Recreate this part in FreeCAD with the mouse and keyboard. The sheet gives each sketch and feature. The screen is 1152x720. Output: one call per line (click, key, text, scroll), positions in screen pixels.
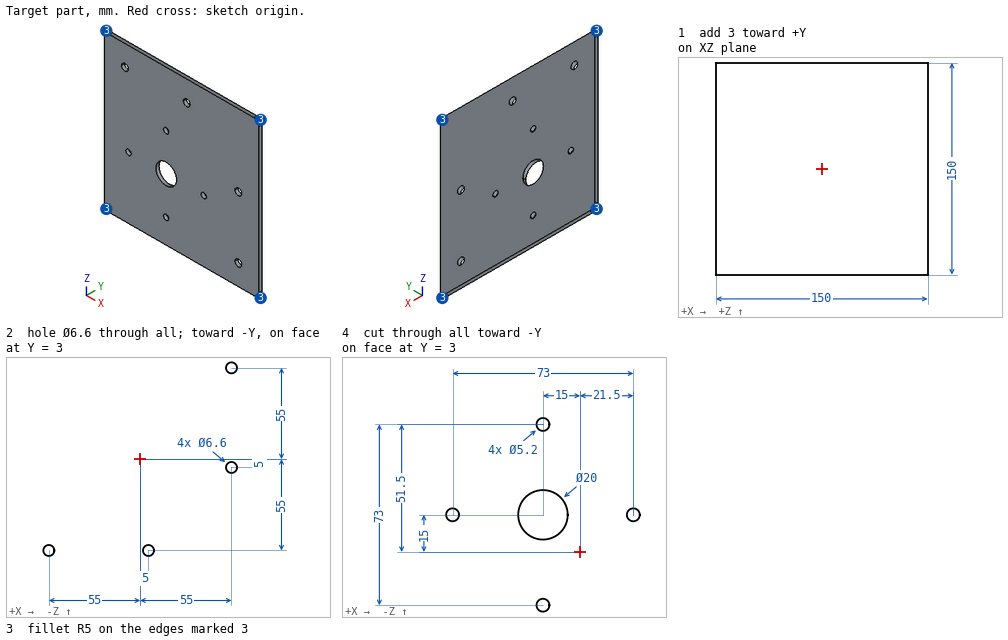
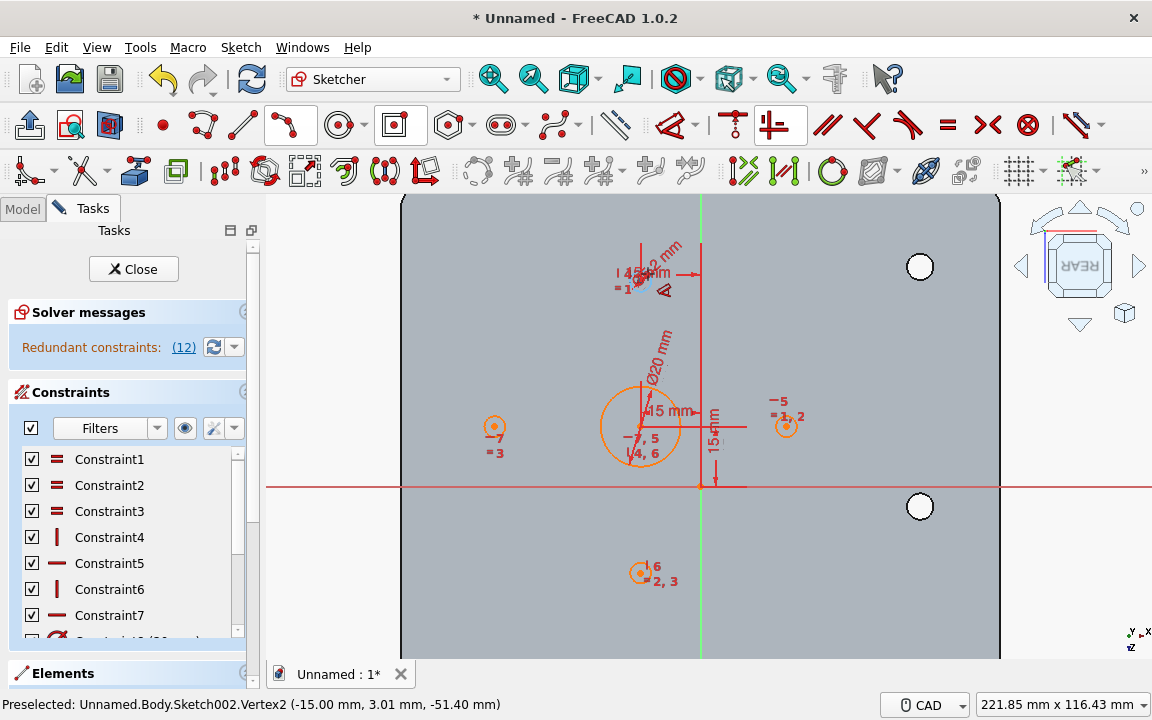
click(641, 573)
click(675, 325)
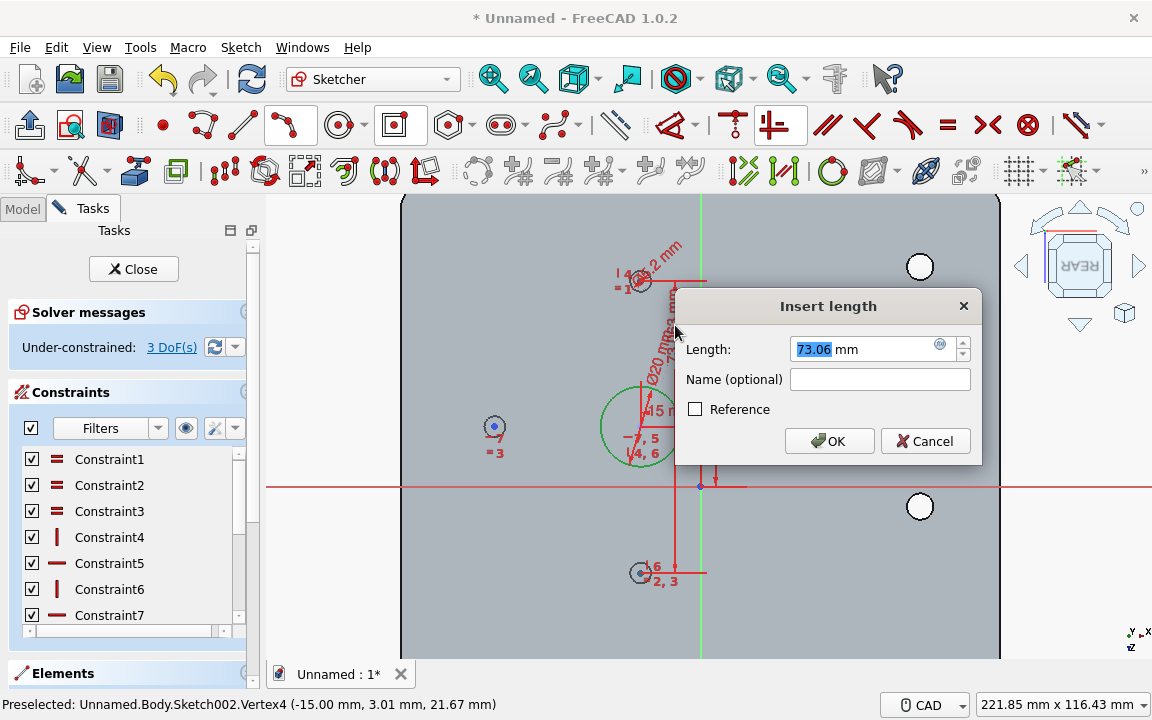
text(73)
key(Return)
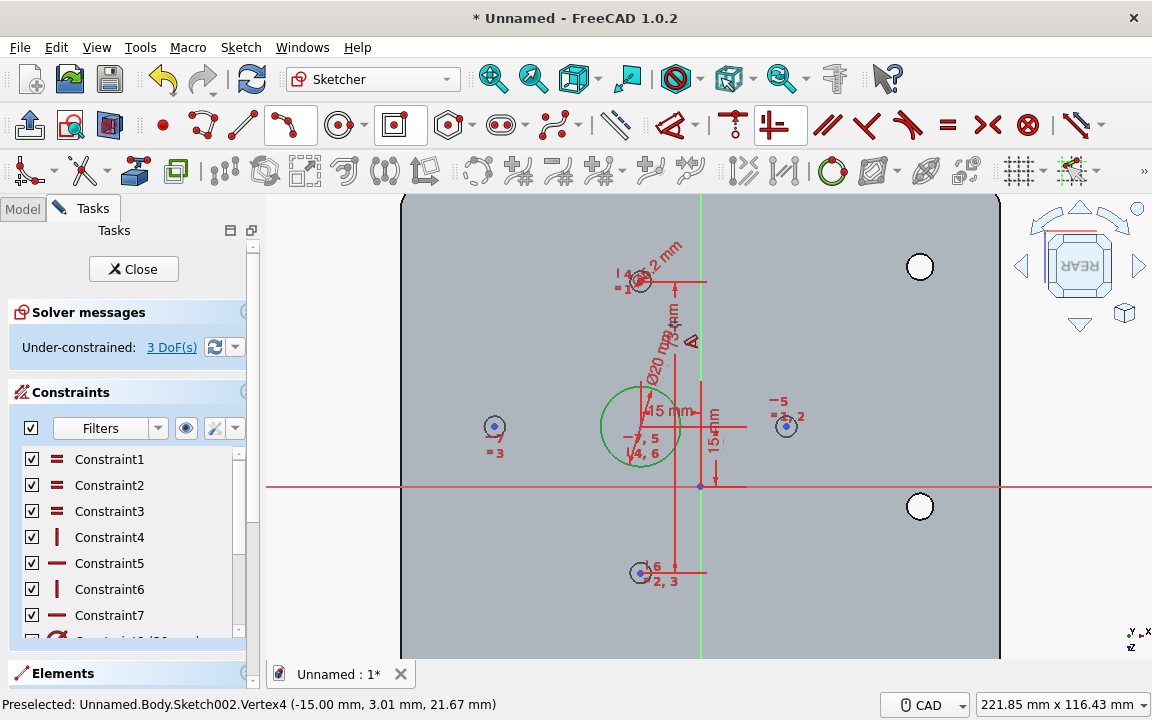
click(786, 427)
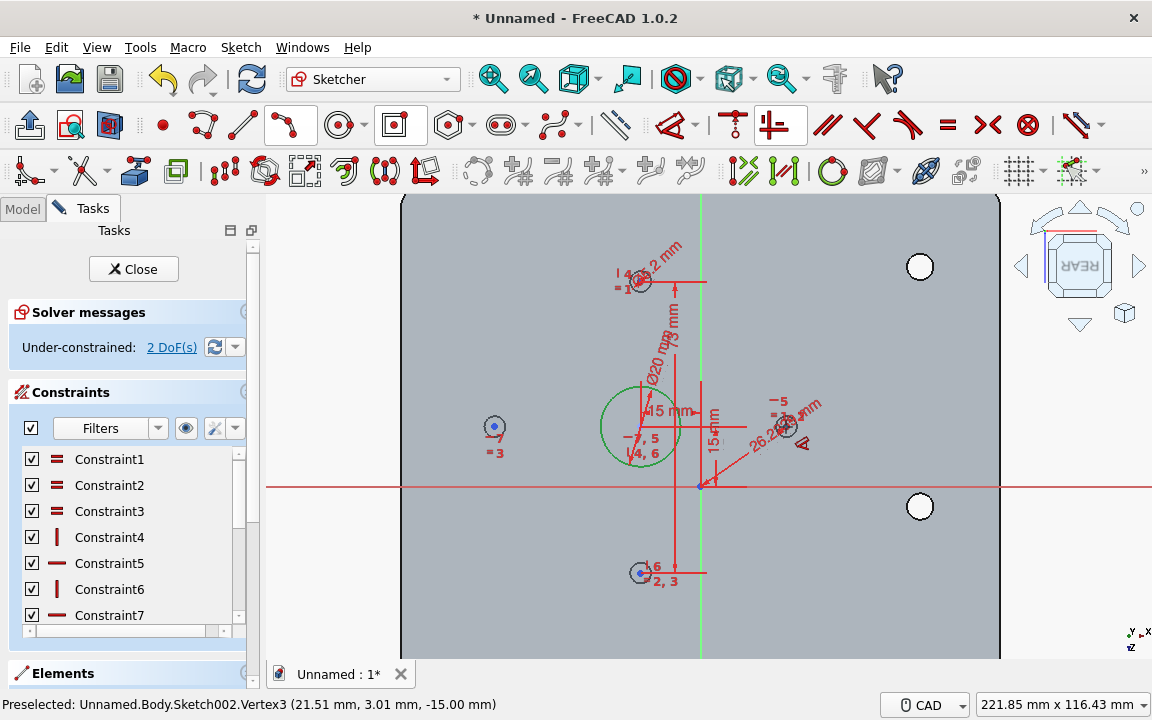
click(495, 427)
click(574, 461)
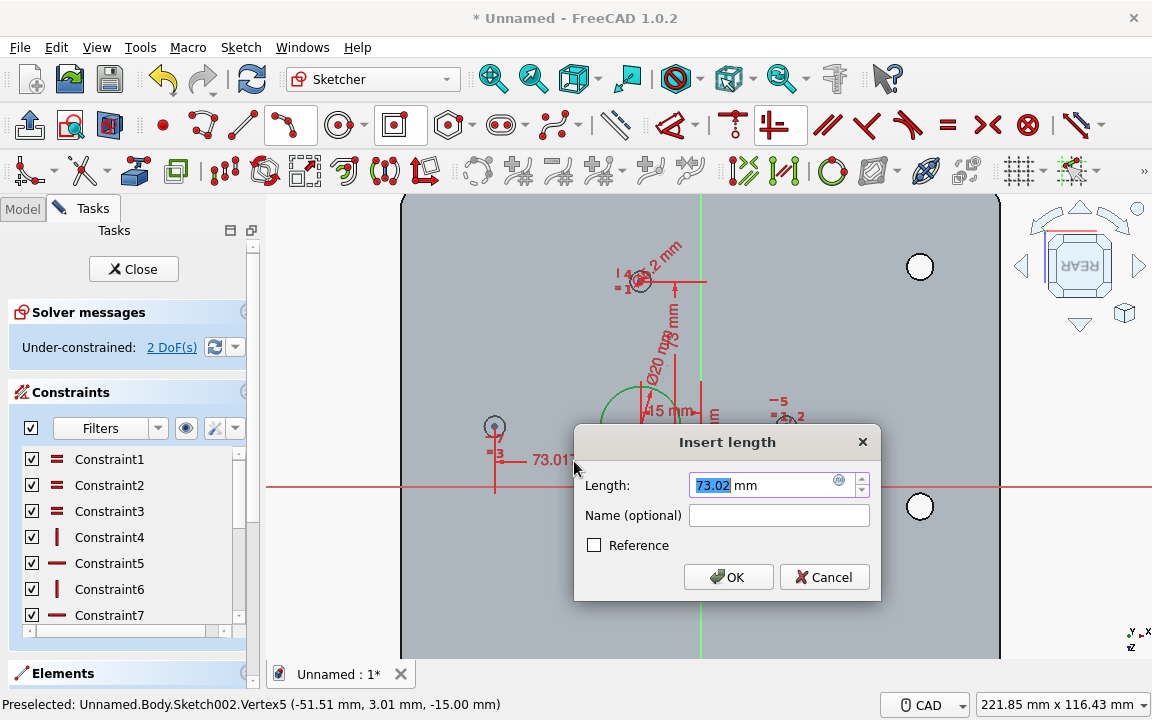
text(73)
key(Return)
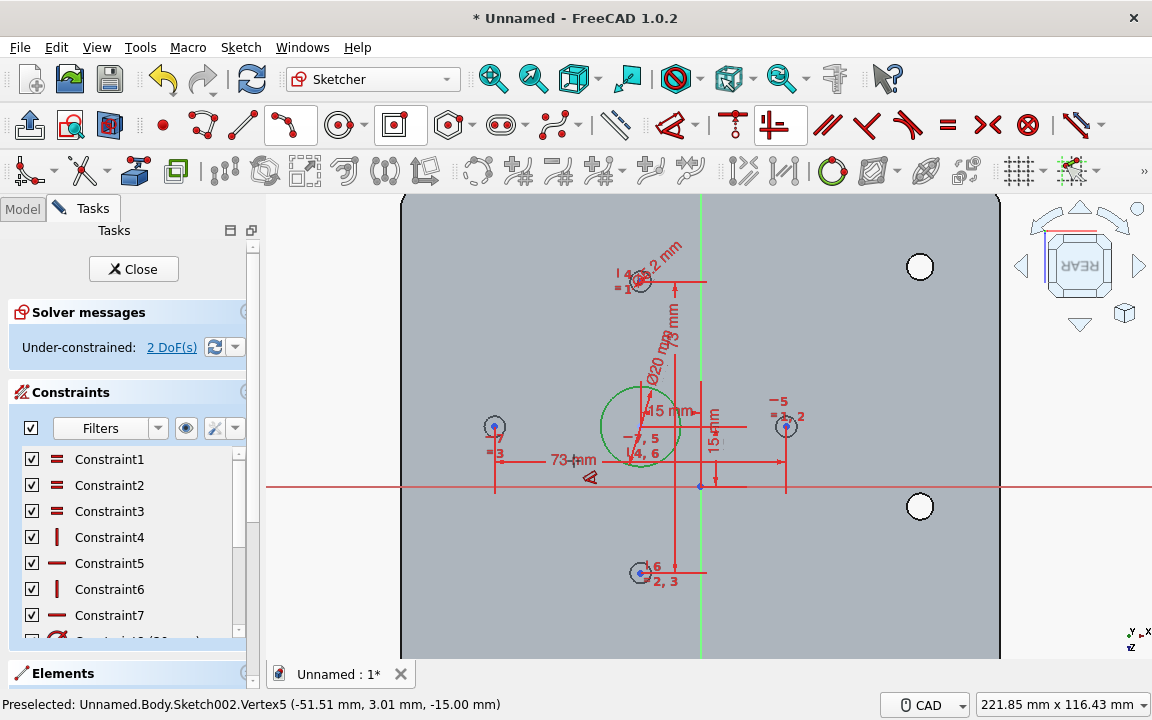
click(641, 282)
click(735, 384)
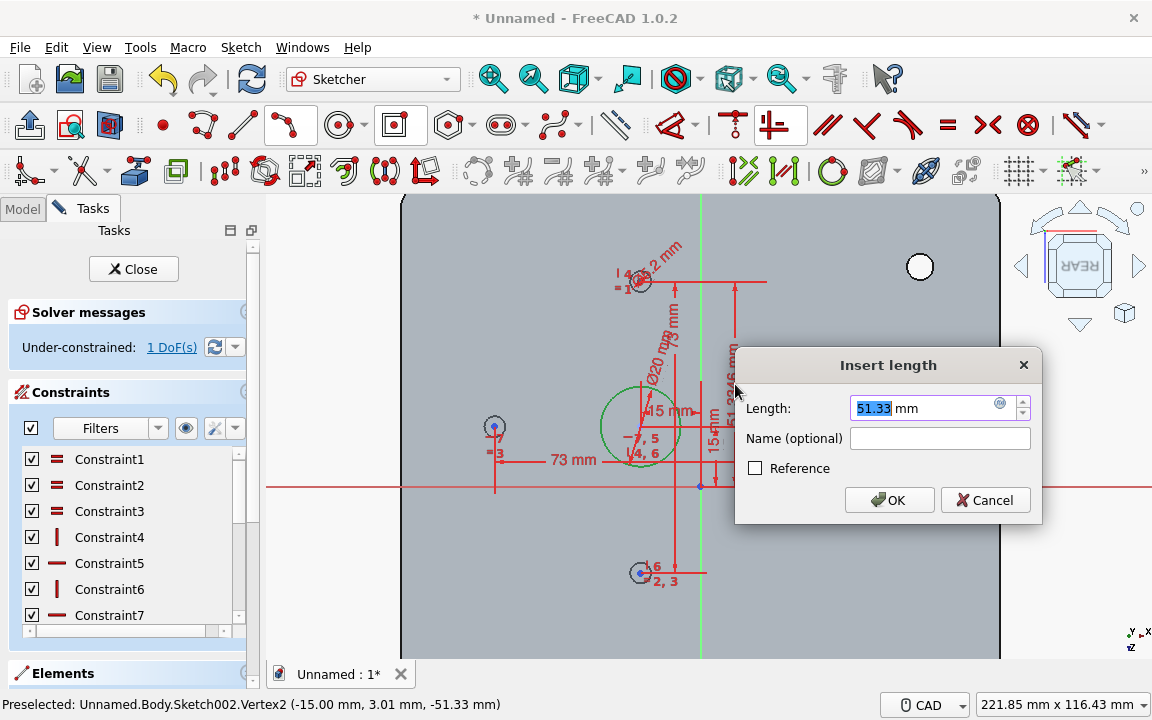
text(51.5)
key(Return)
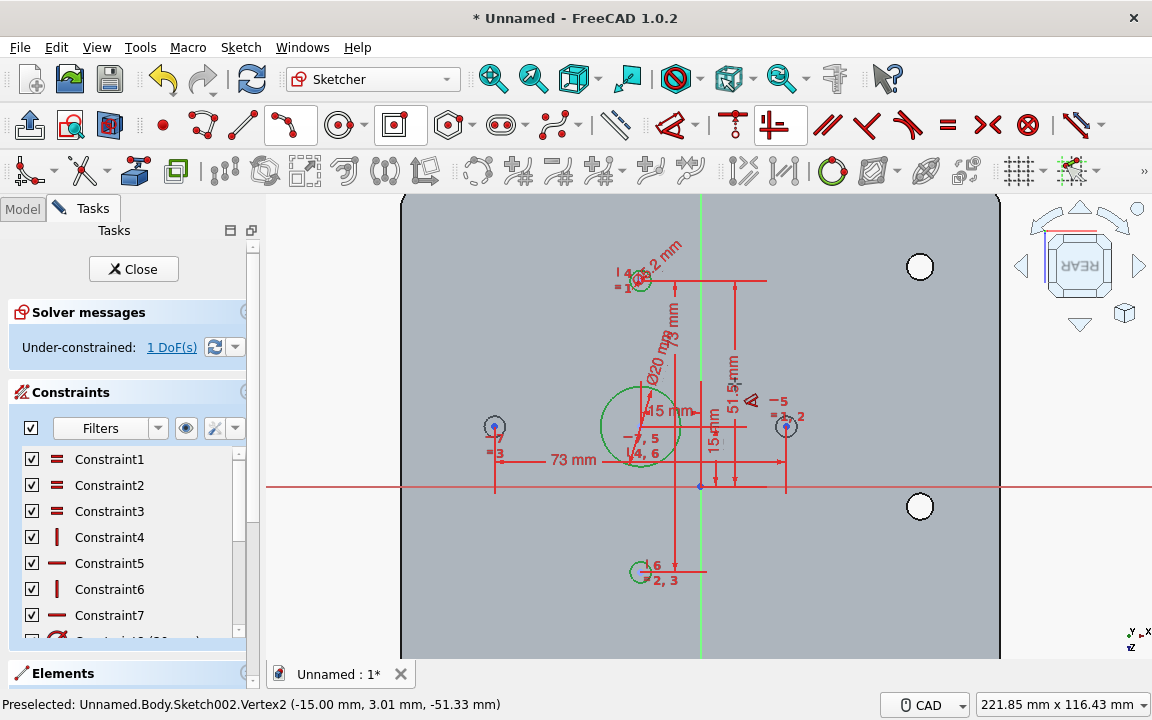
click(786, 427)
click(743, 521)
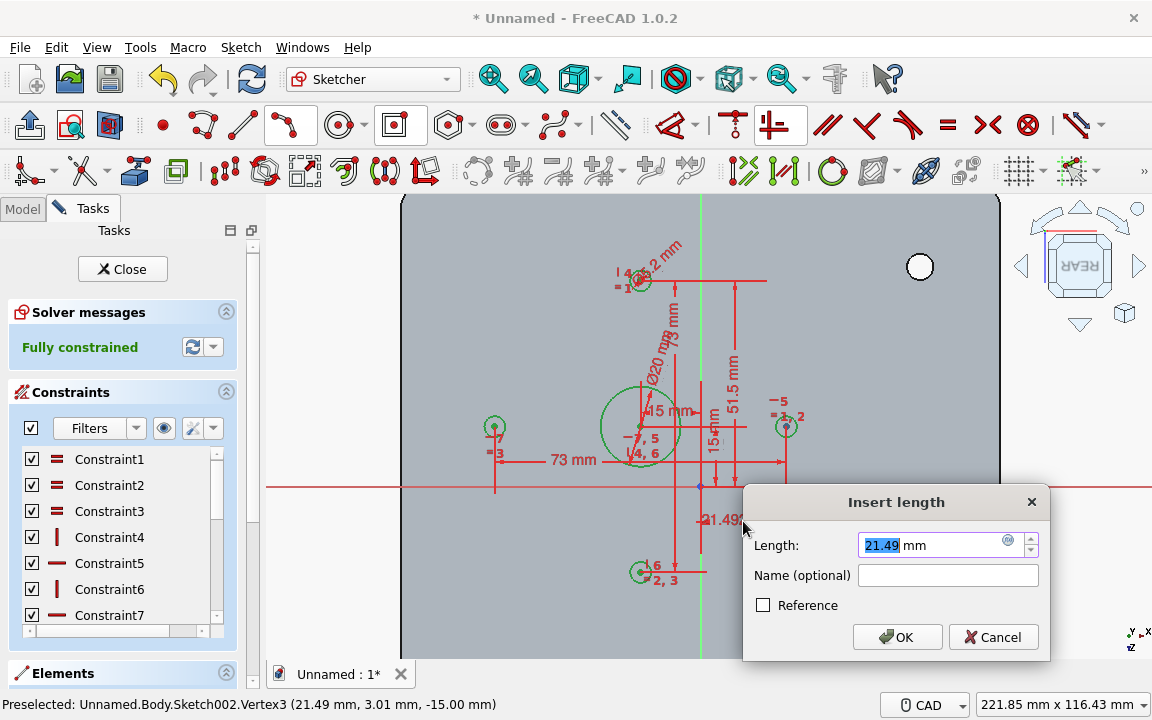
text(21.5)
key(Return)
key(Escape)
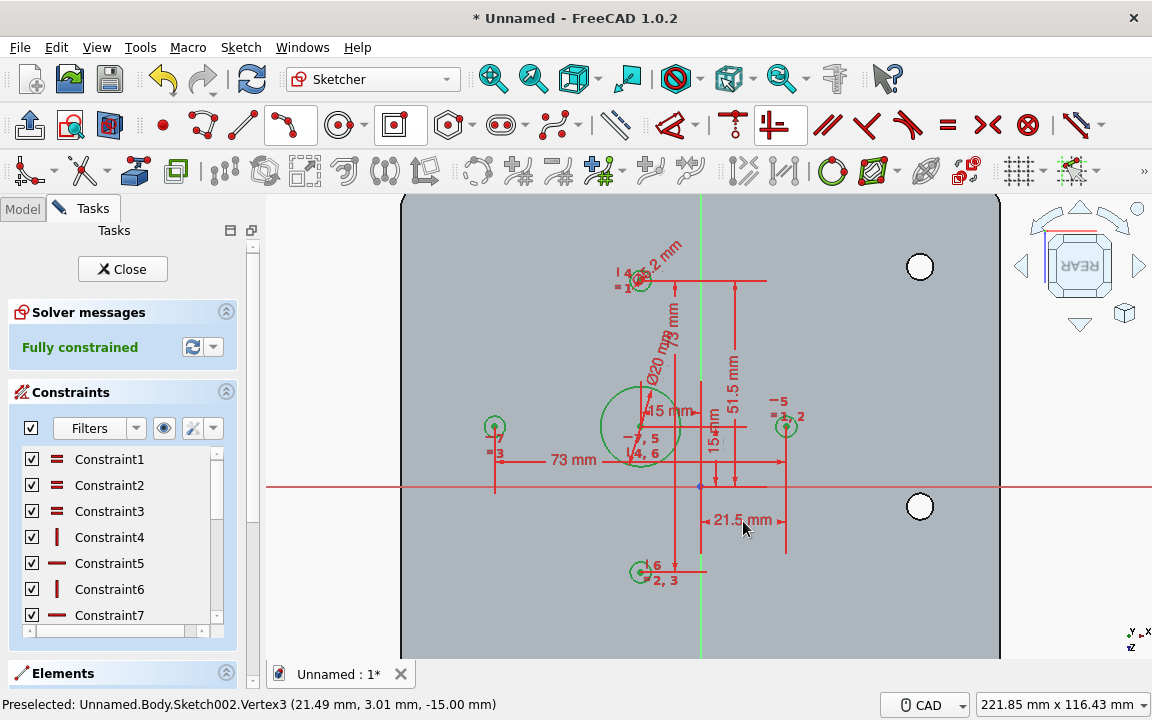
click(123, 269)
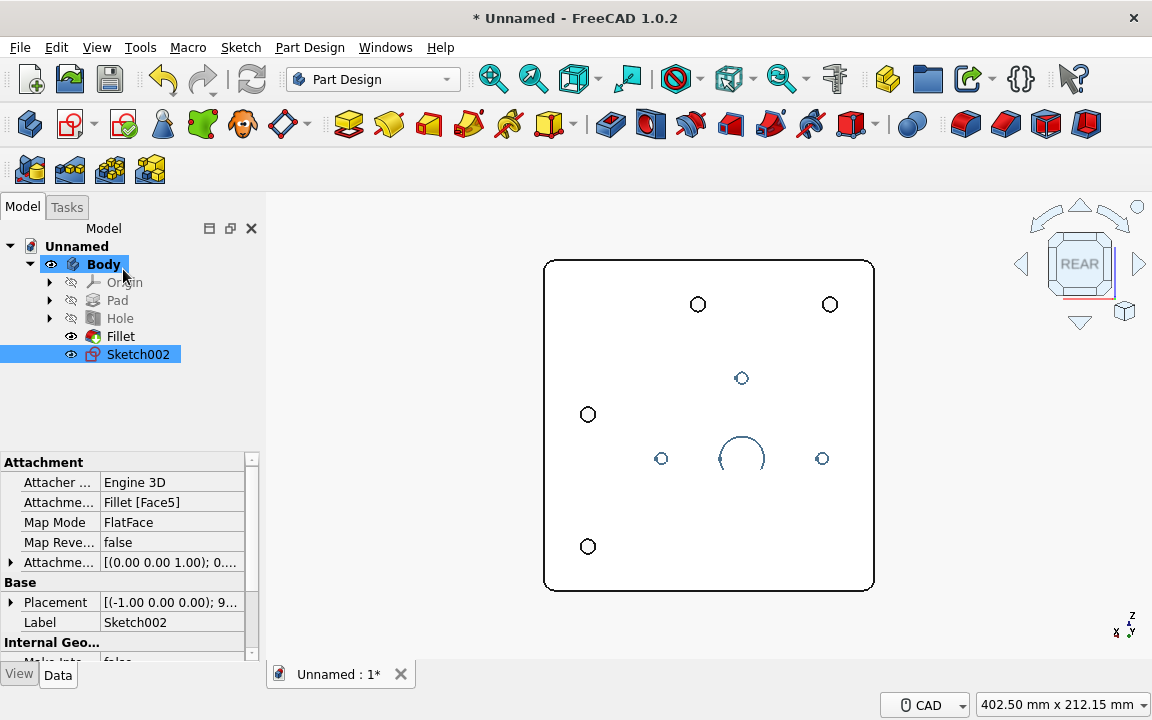
click(612, 124)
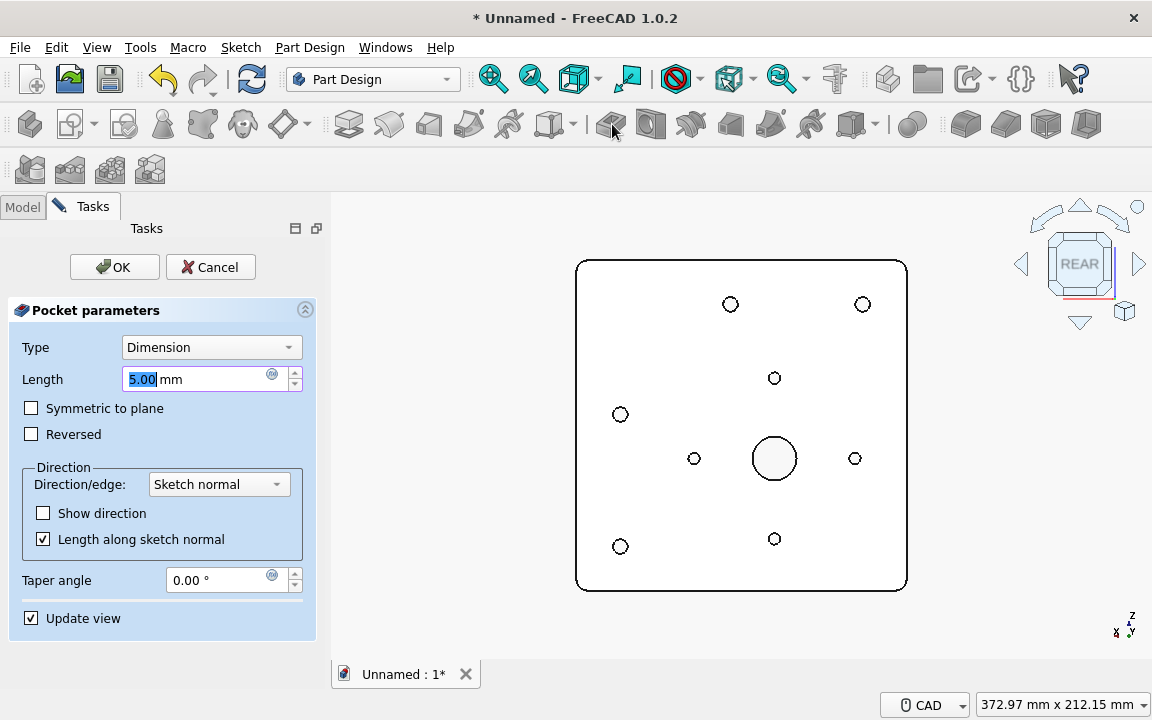
click(212, 348)